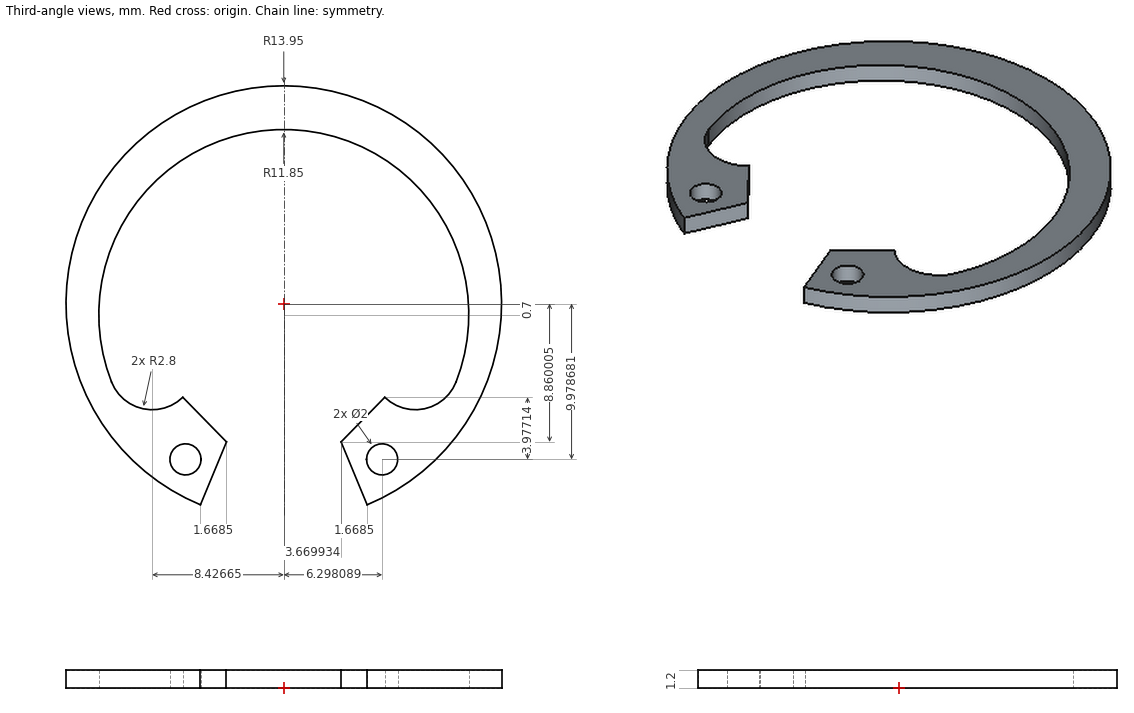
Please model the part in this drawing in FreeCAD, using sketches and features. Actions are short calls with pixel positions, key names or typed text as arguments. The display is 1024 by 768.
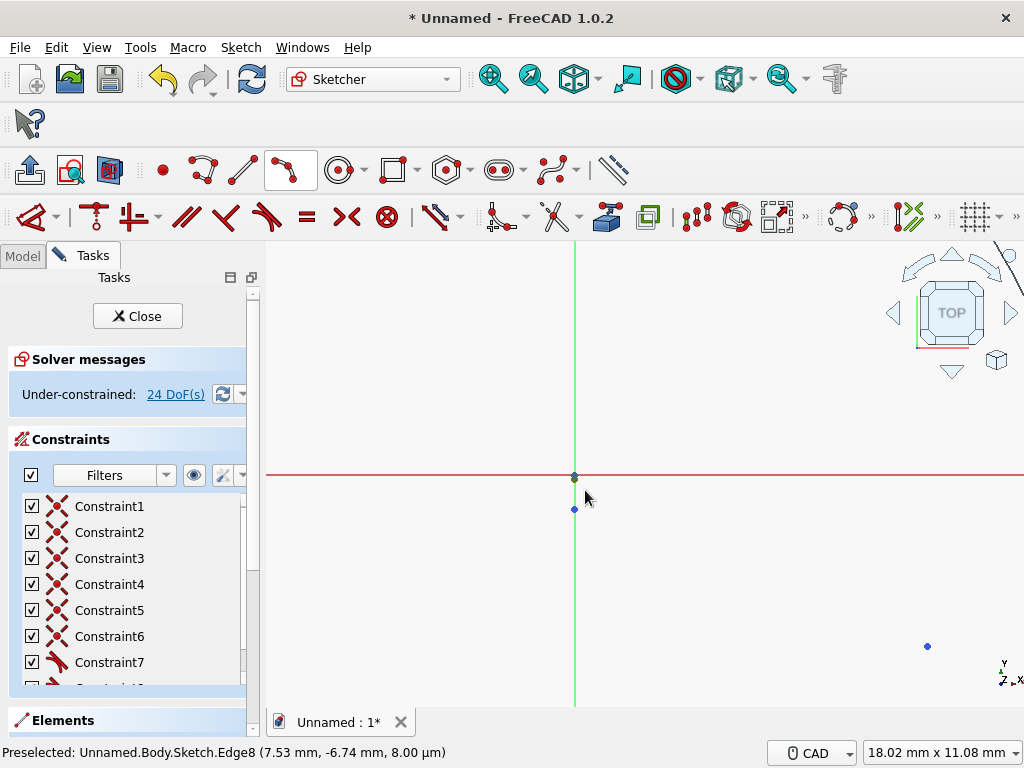
click(94, 218)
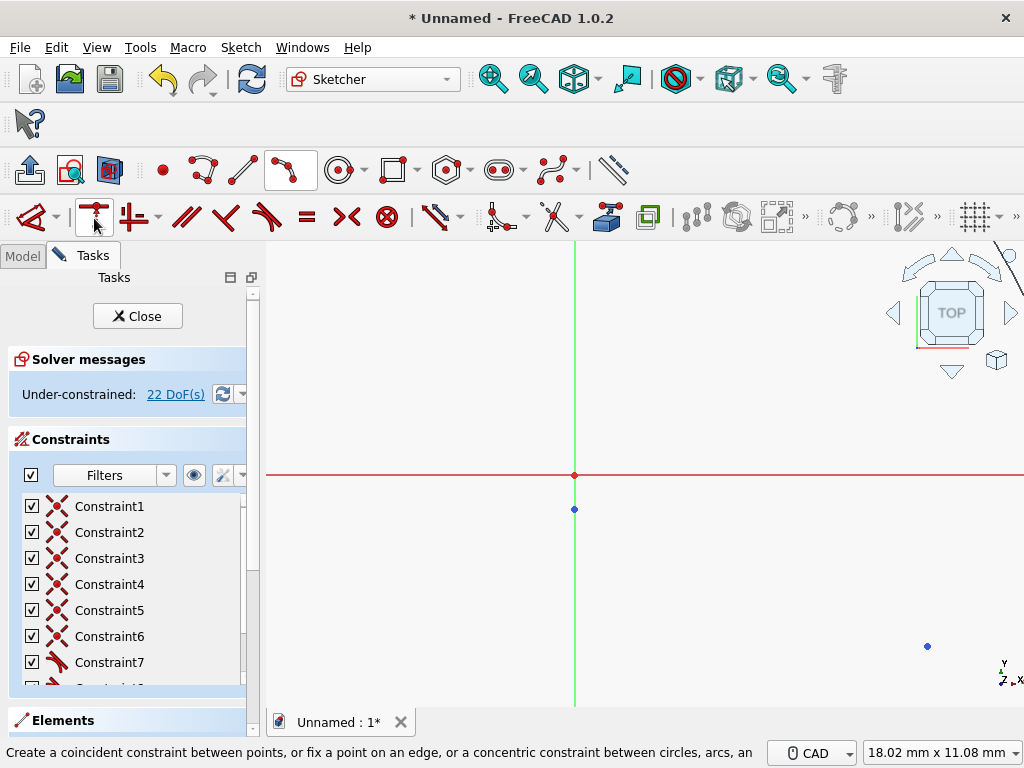
scroll(577, 481, down, 7)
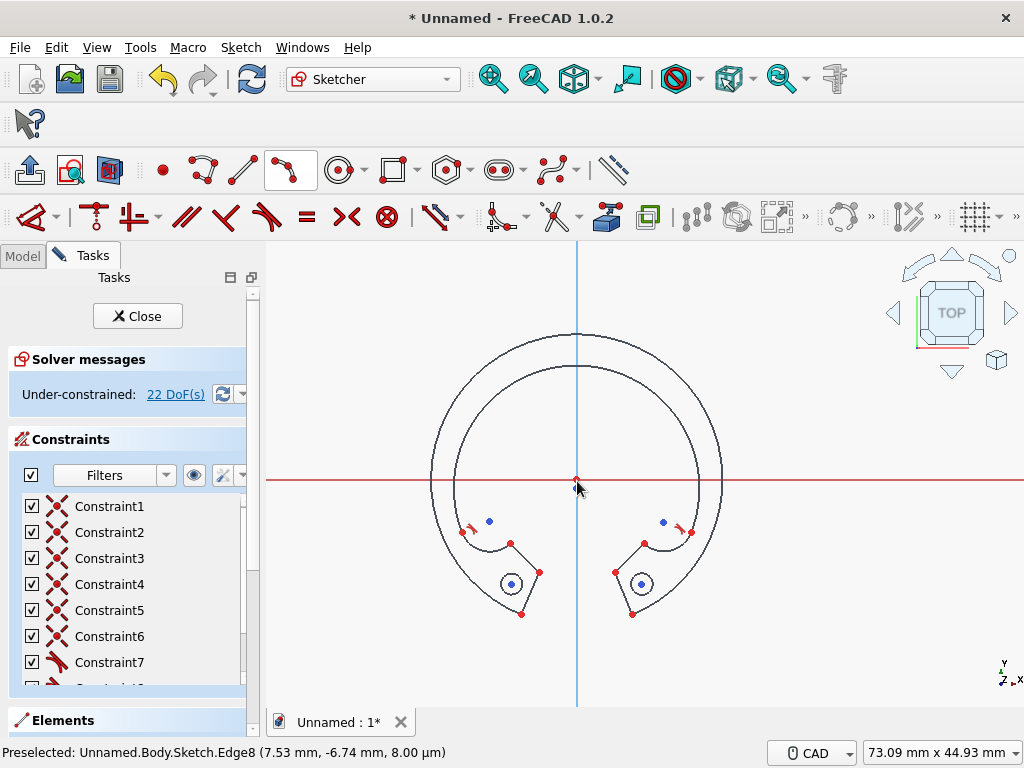
click(473, 546)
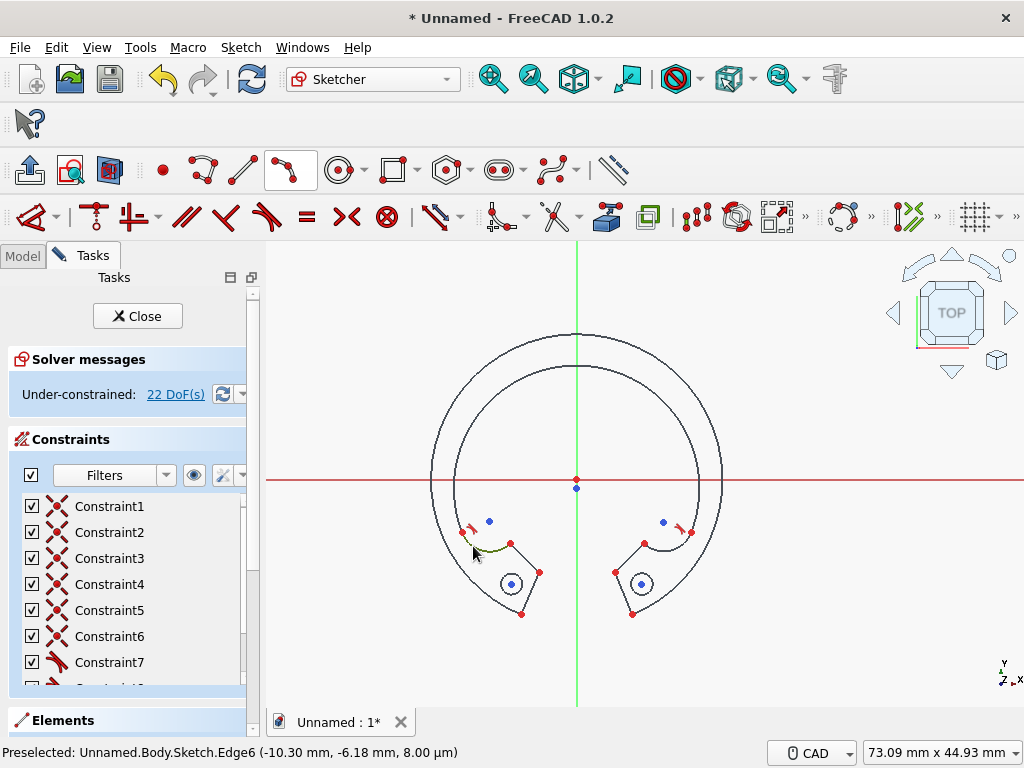
click(659, 551)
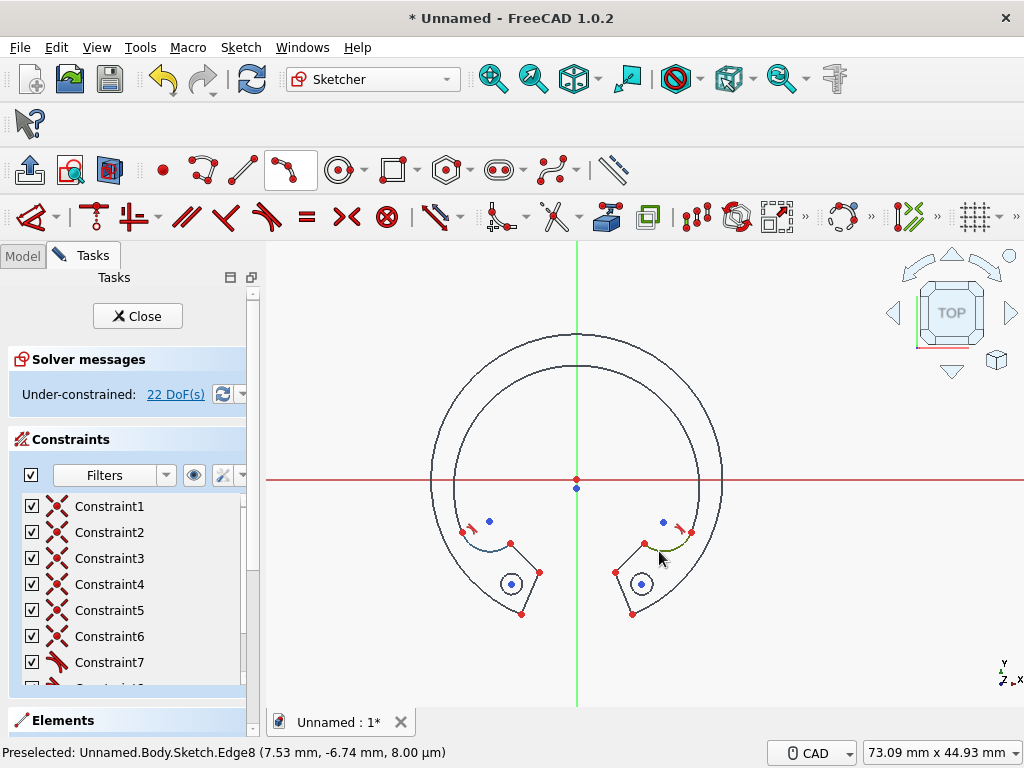
click(308, 218)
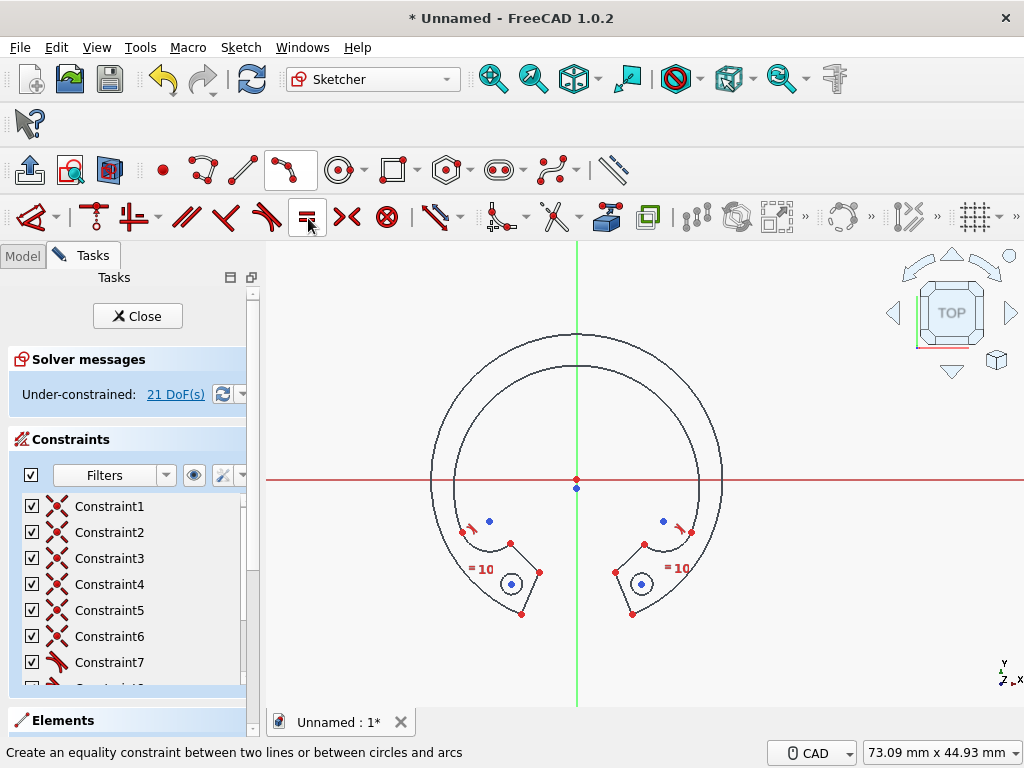
scroll(650, 576, up, 2)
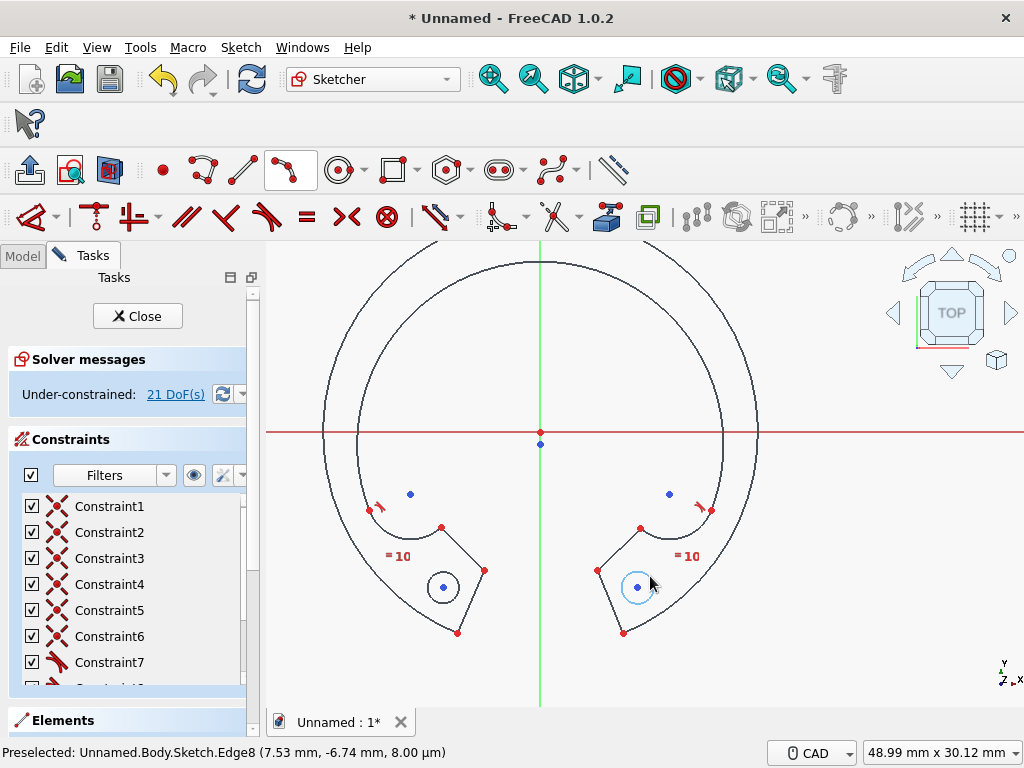
click(649, 576)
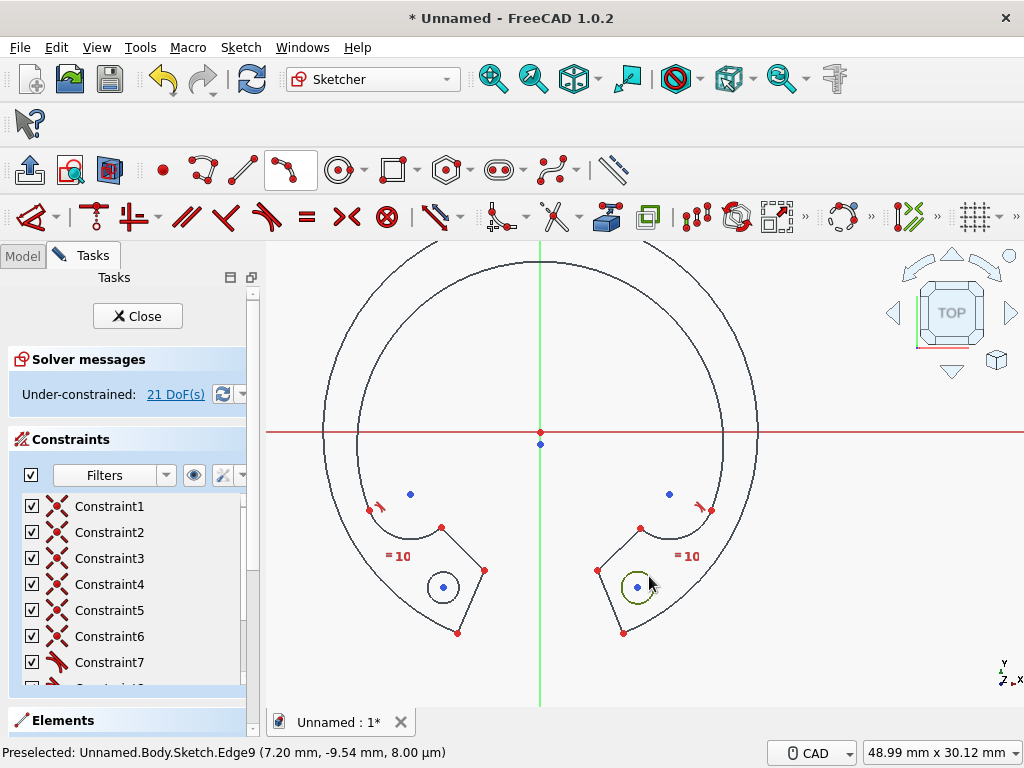
click(454, 577)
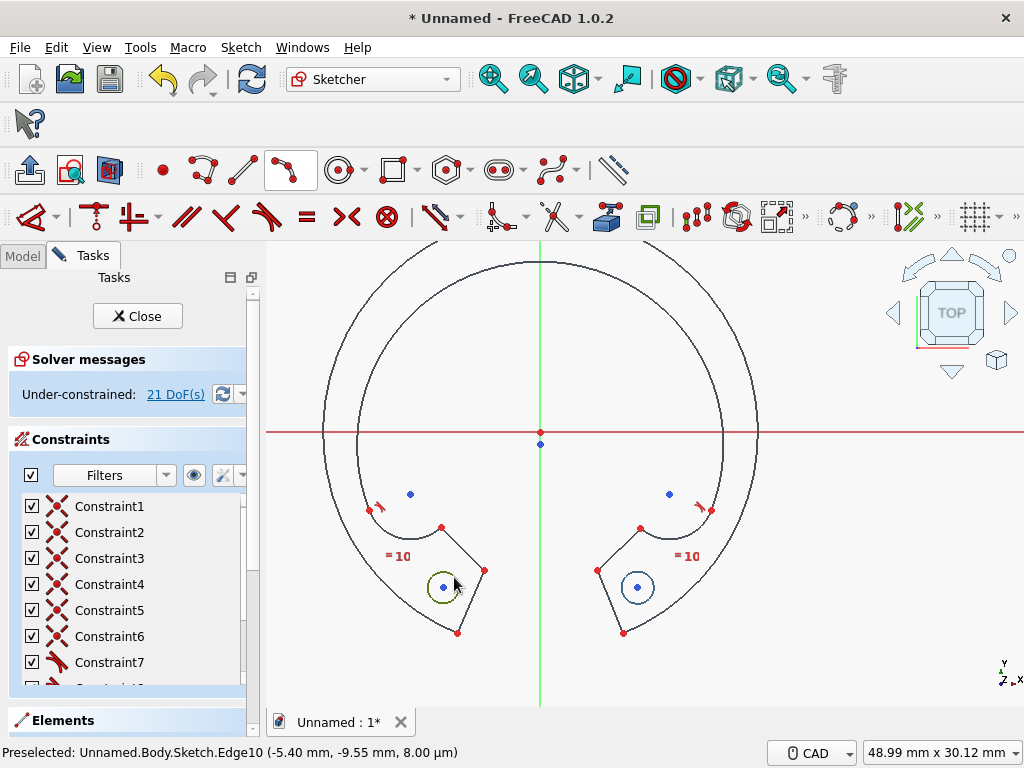
click(308, 218)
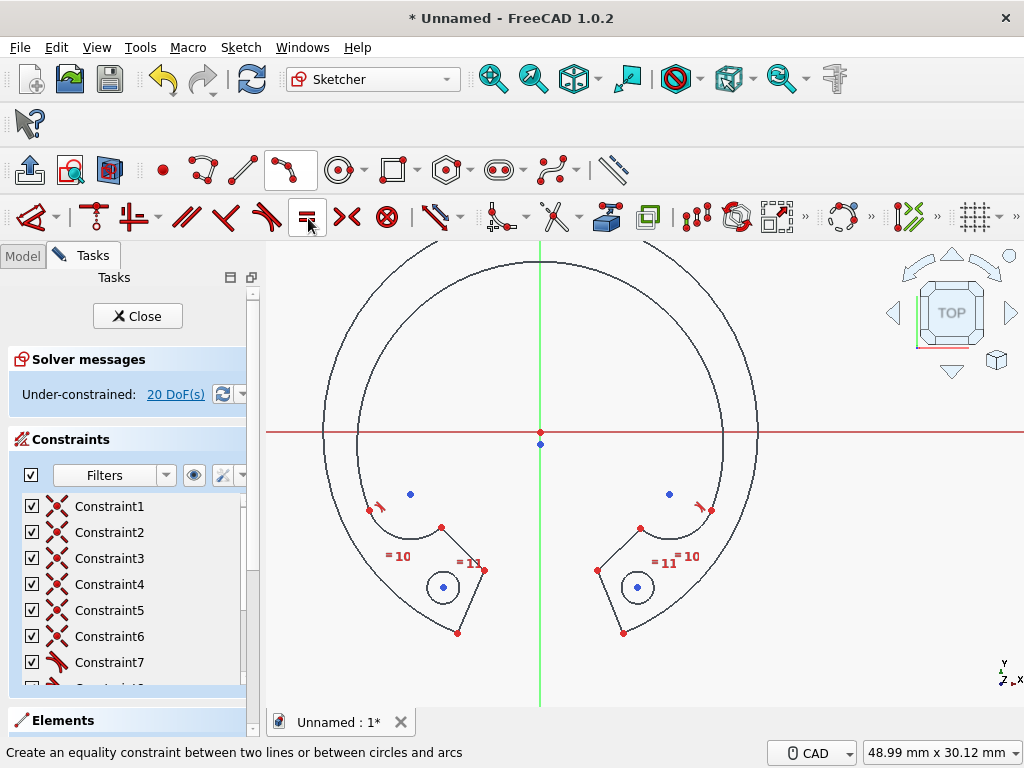
click(540, 445)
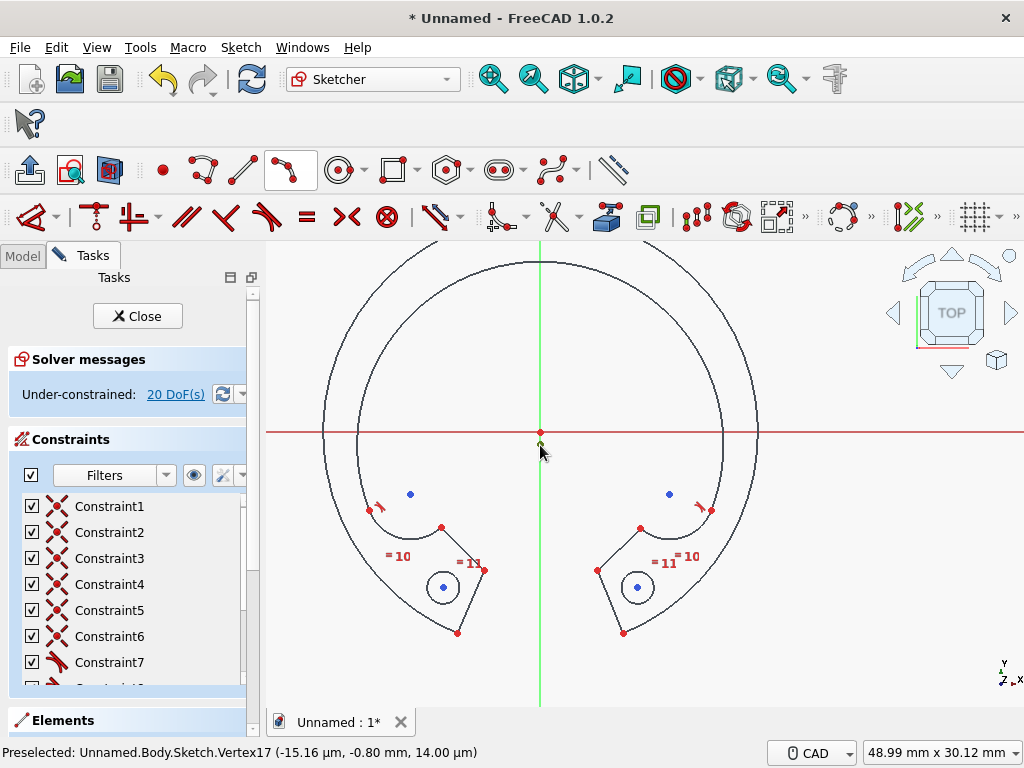
click(541, 650)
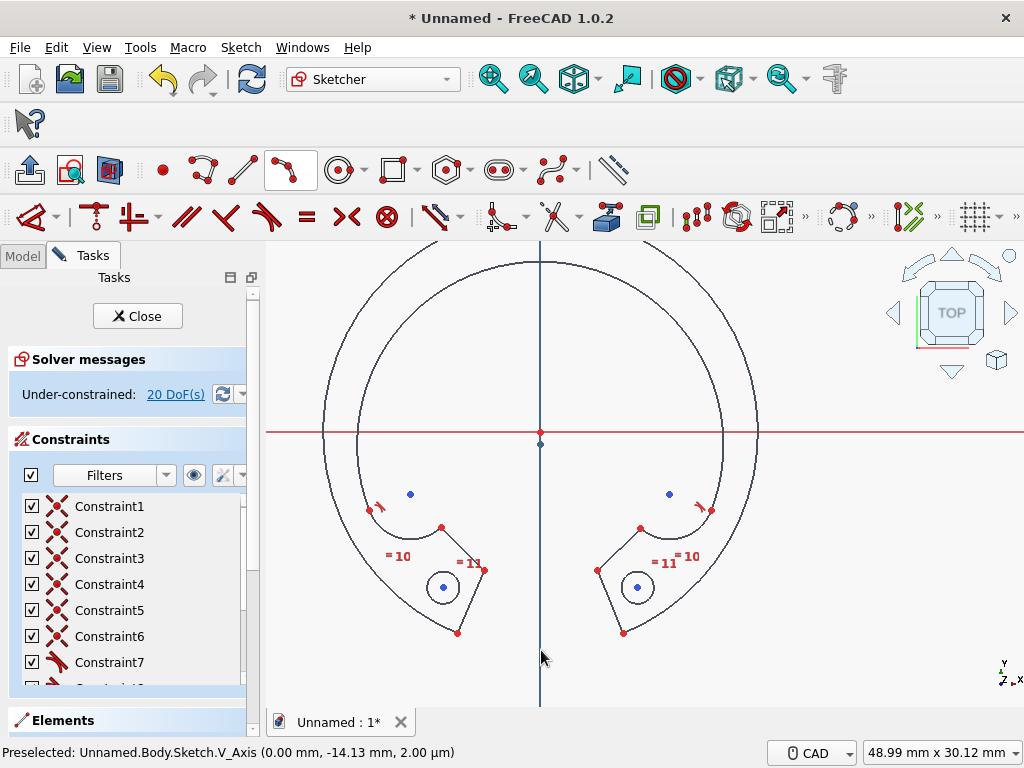
click(94, 218)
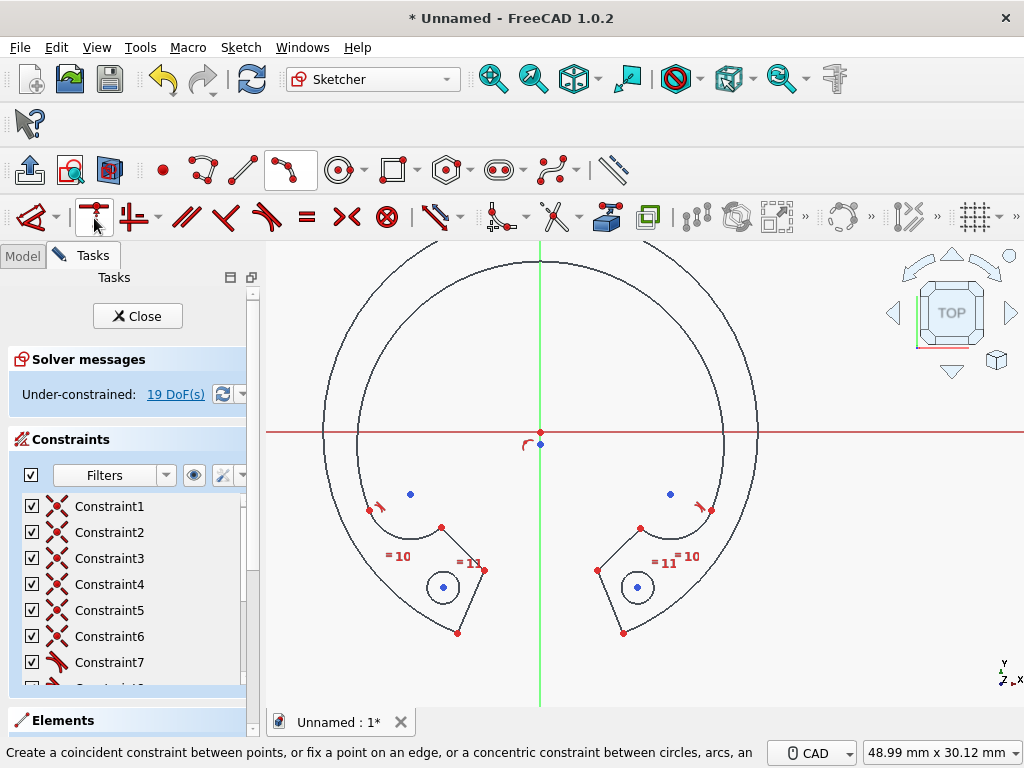
click(638, 588)